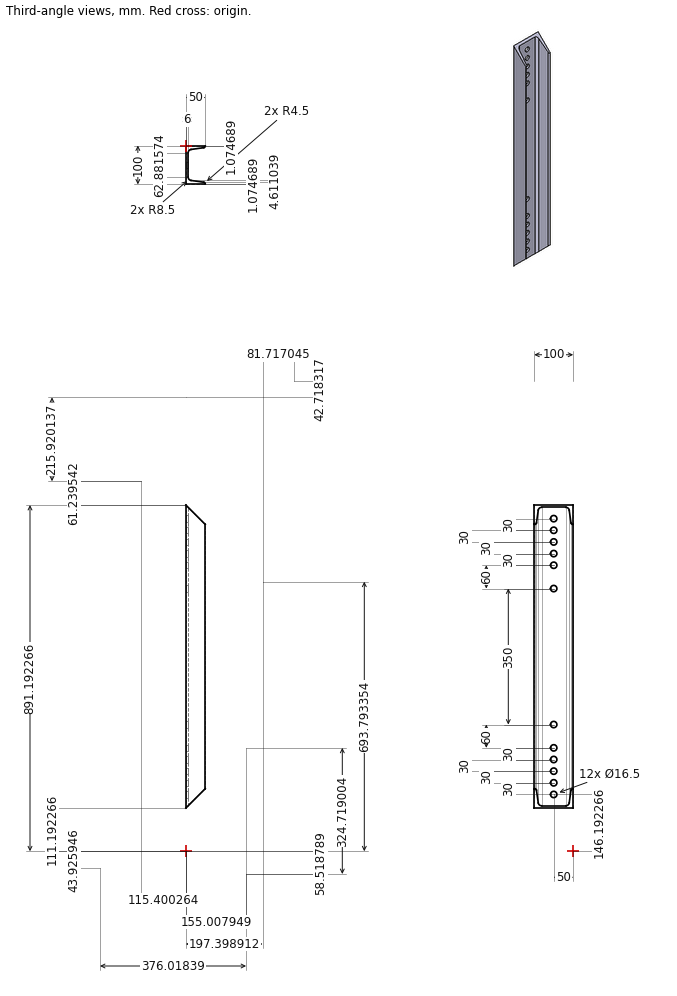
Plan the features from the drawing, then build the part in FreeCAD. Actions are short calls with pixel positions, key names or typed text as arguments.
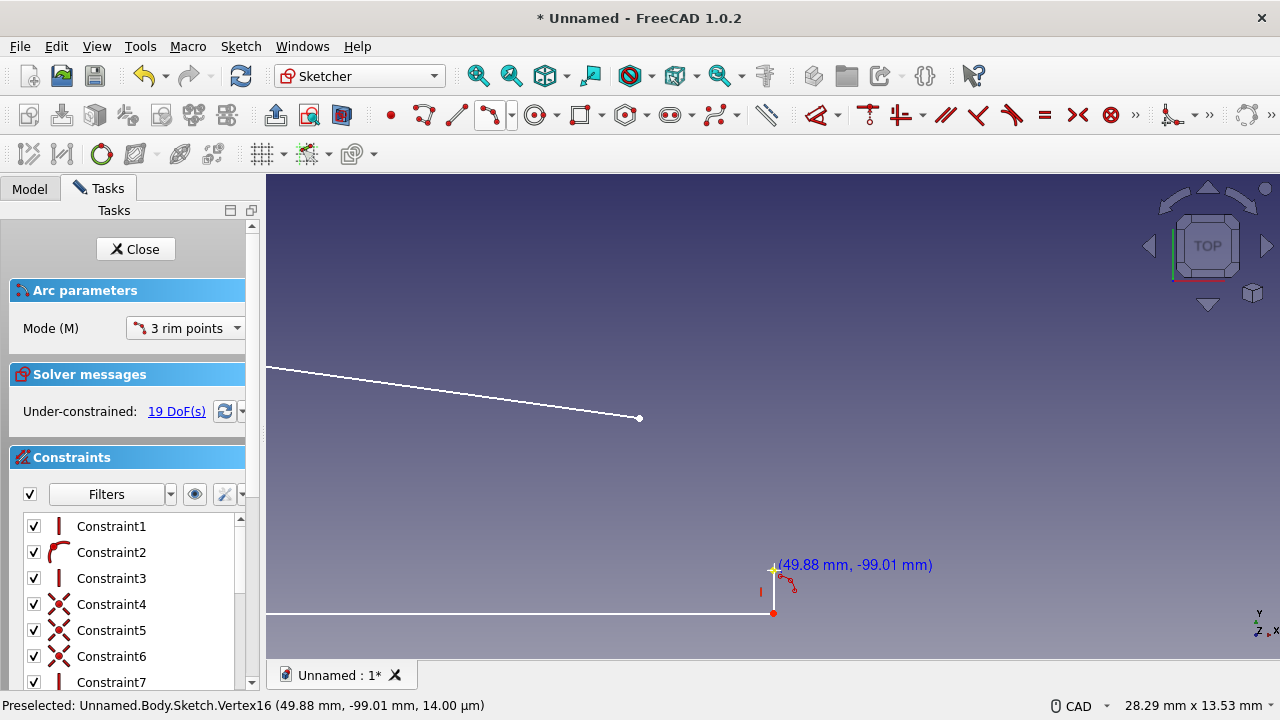
scroll(787, 576, down, 12)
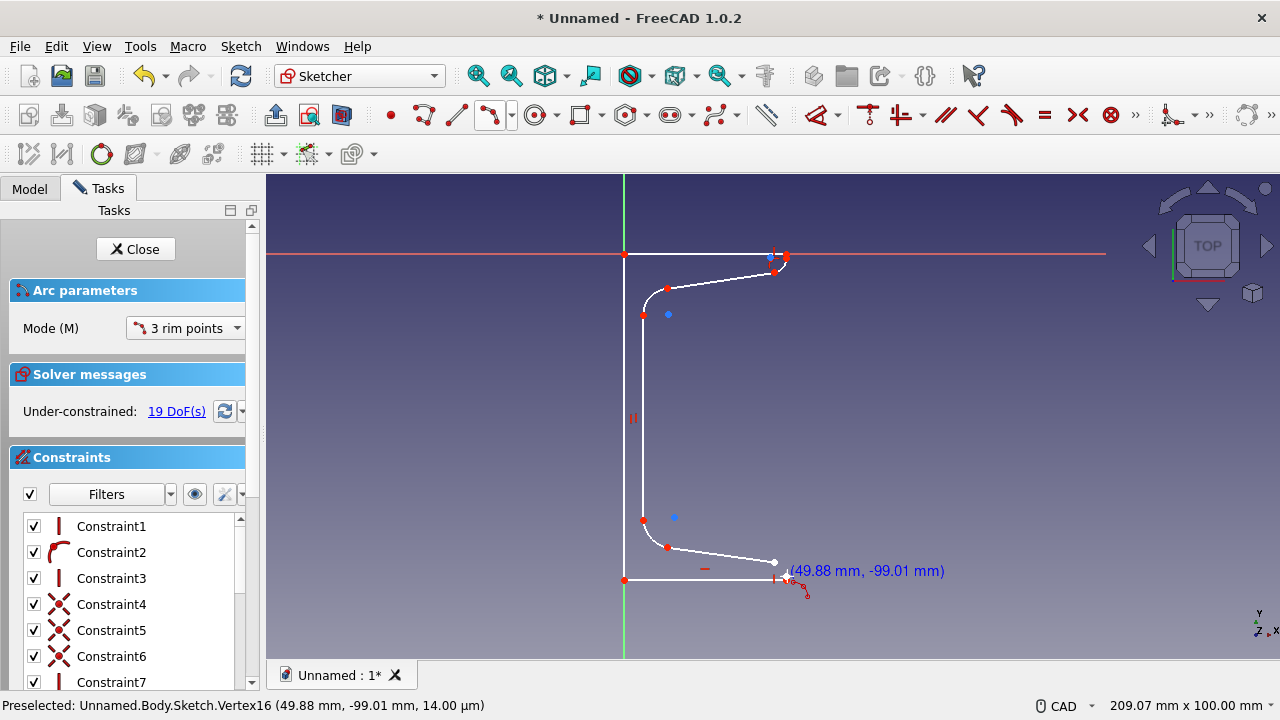
click(774, 562)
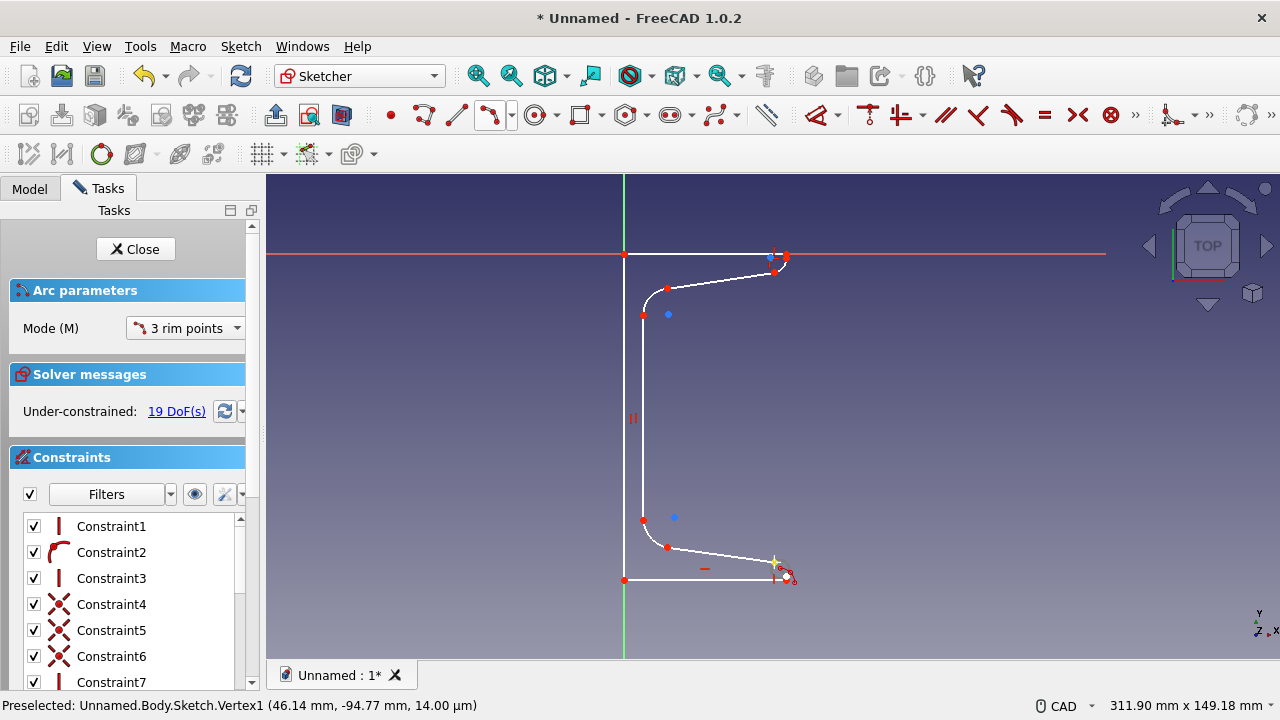
scroll(783, 566, up, 8)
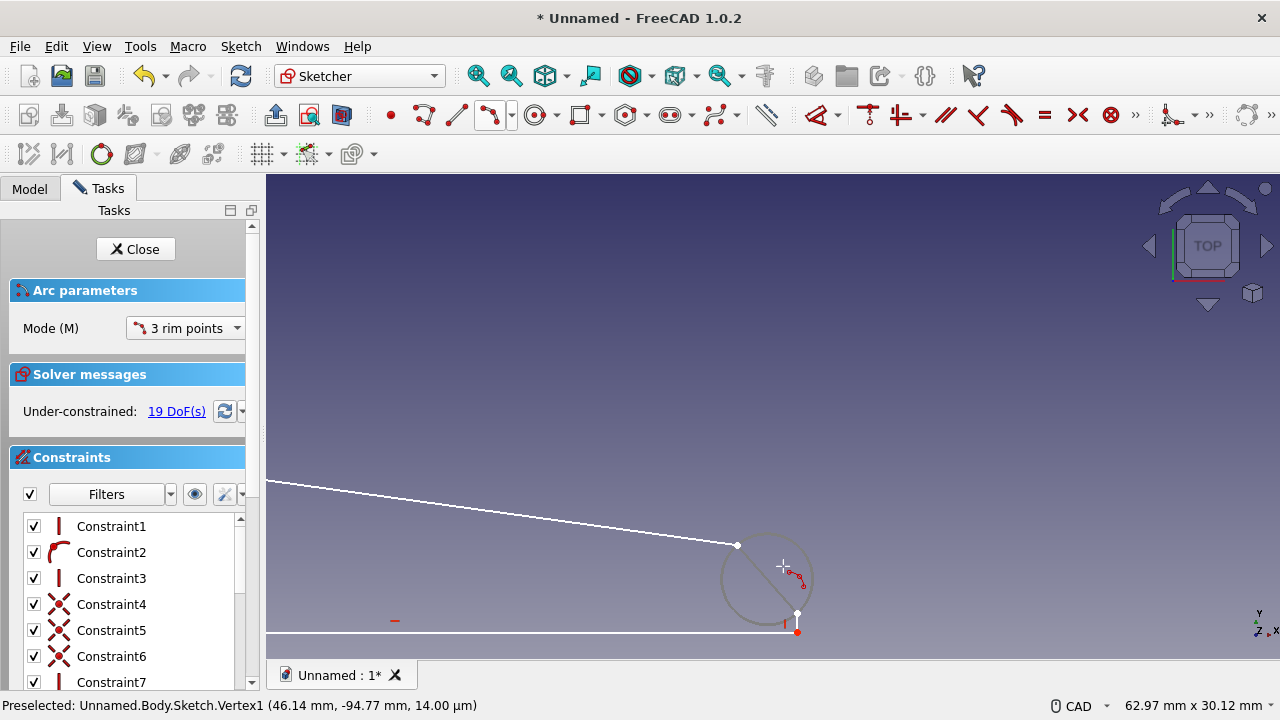
click(781, 565)
key(Escape)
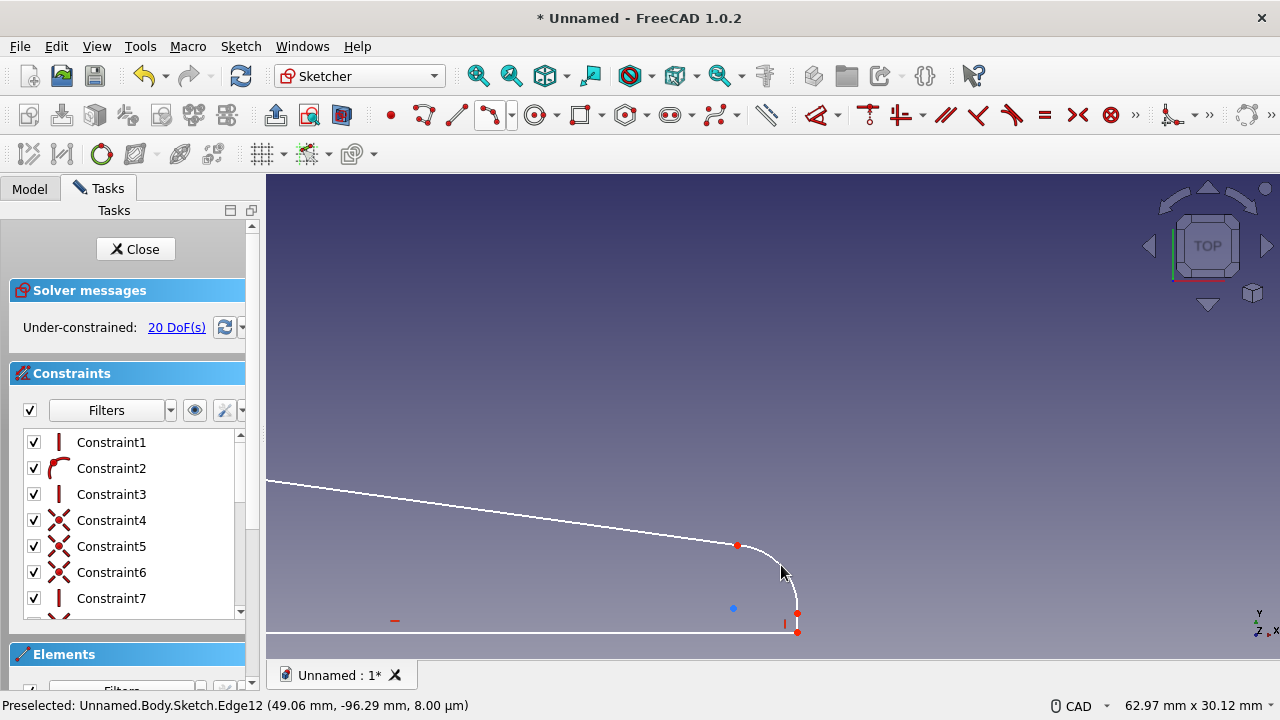
scroll(782, 566, down, 8)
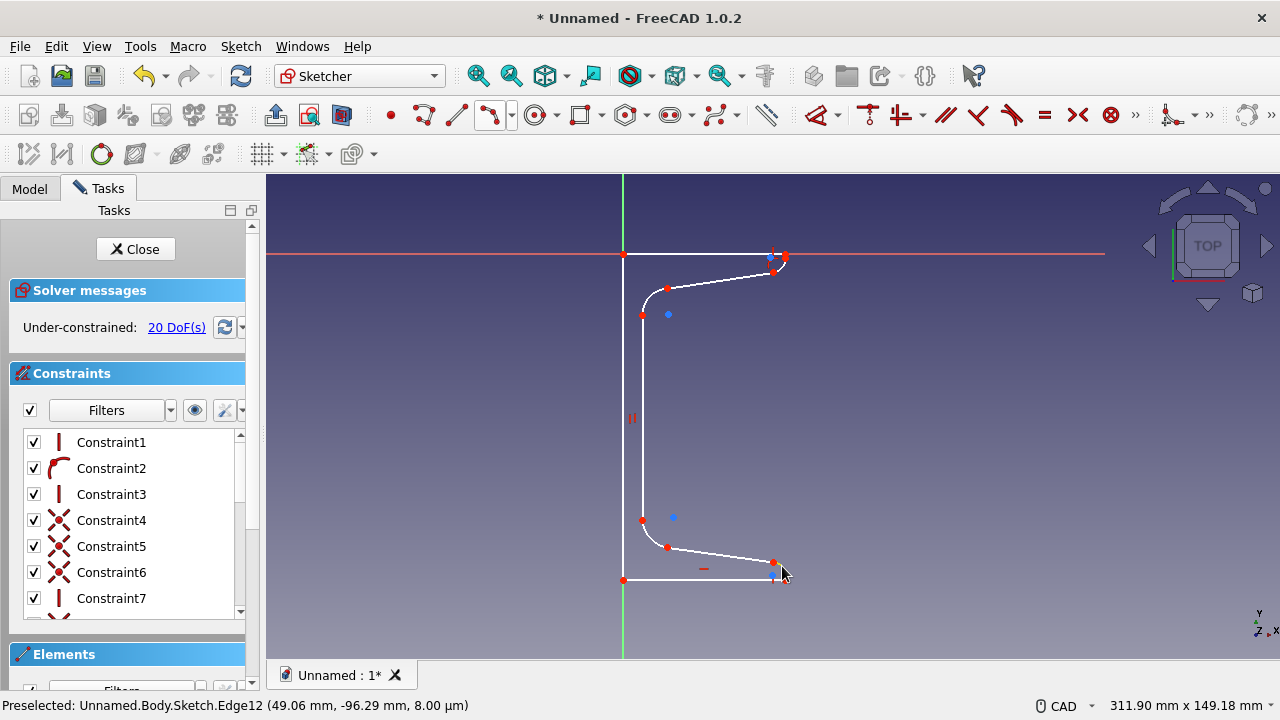
click(741, 558)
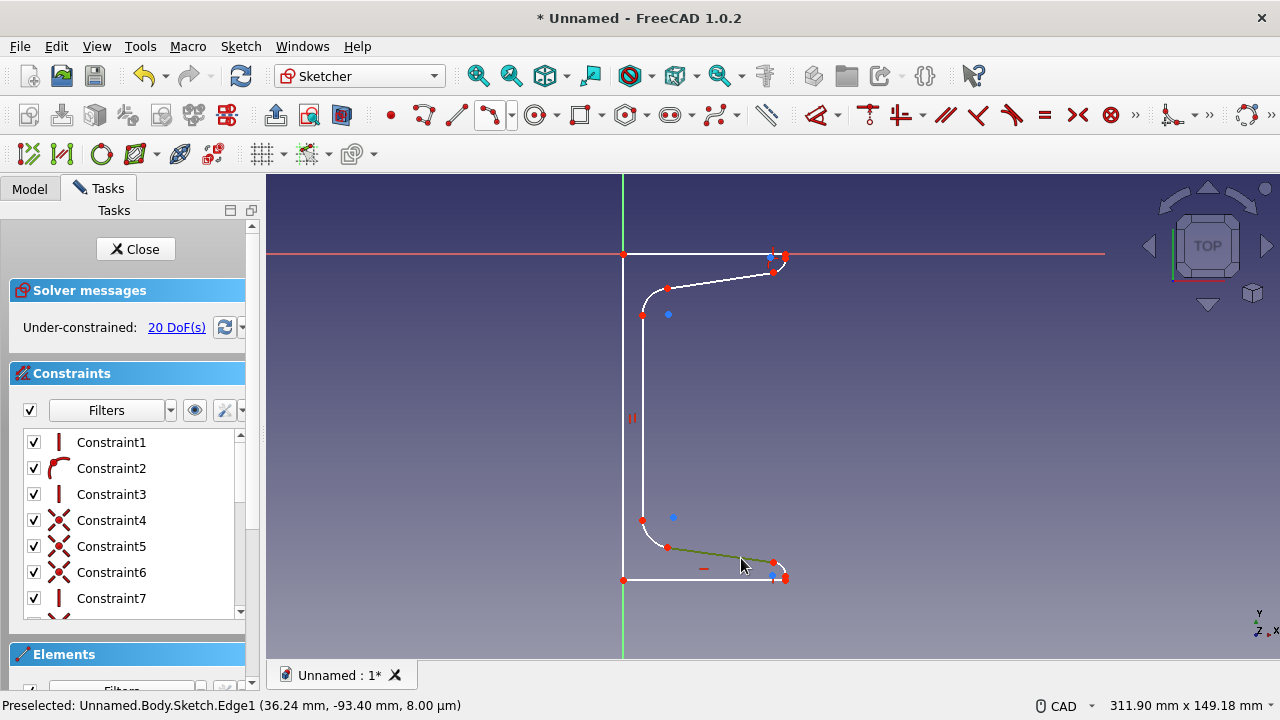
click(646, 532)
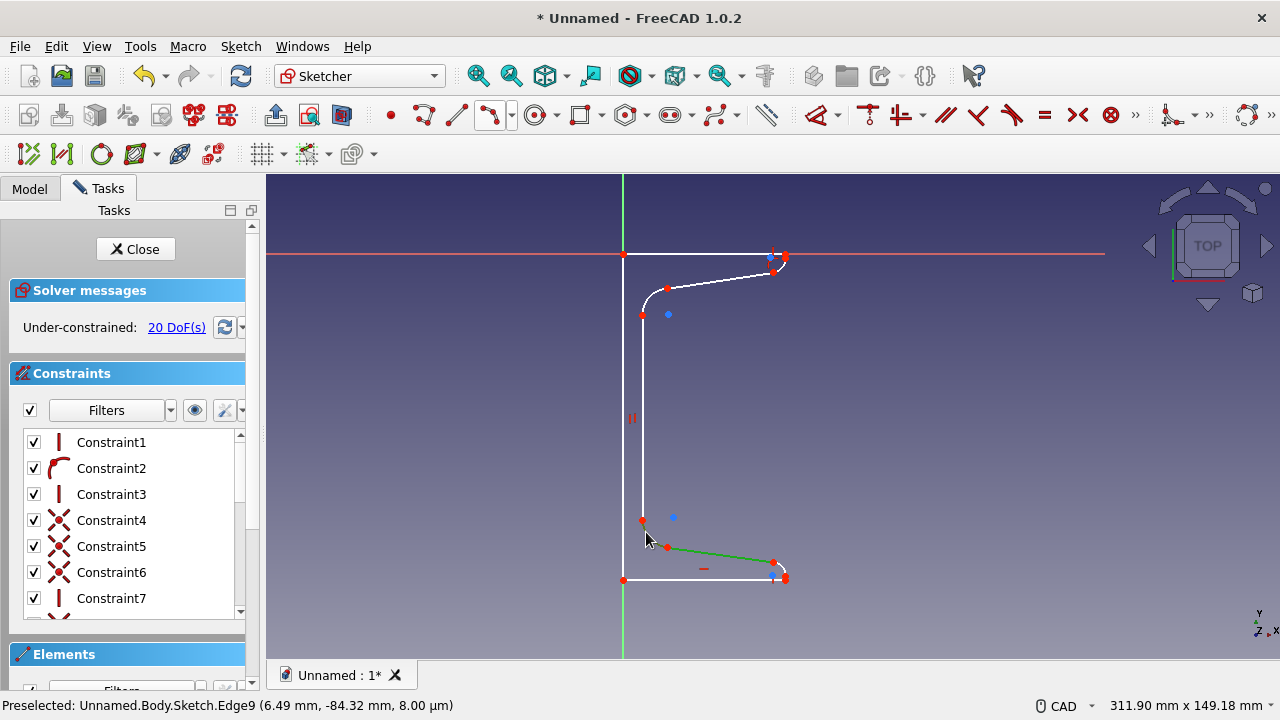
click(1012, 116)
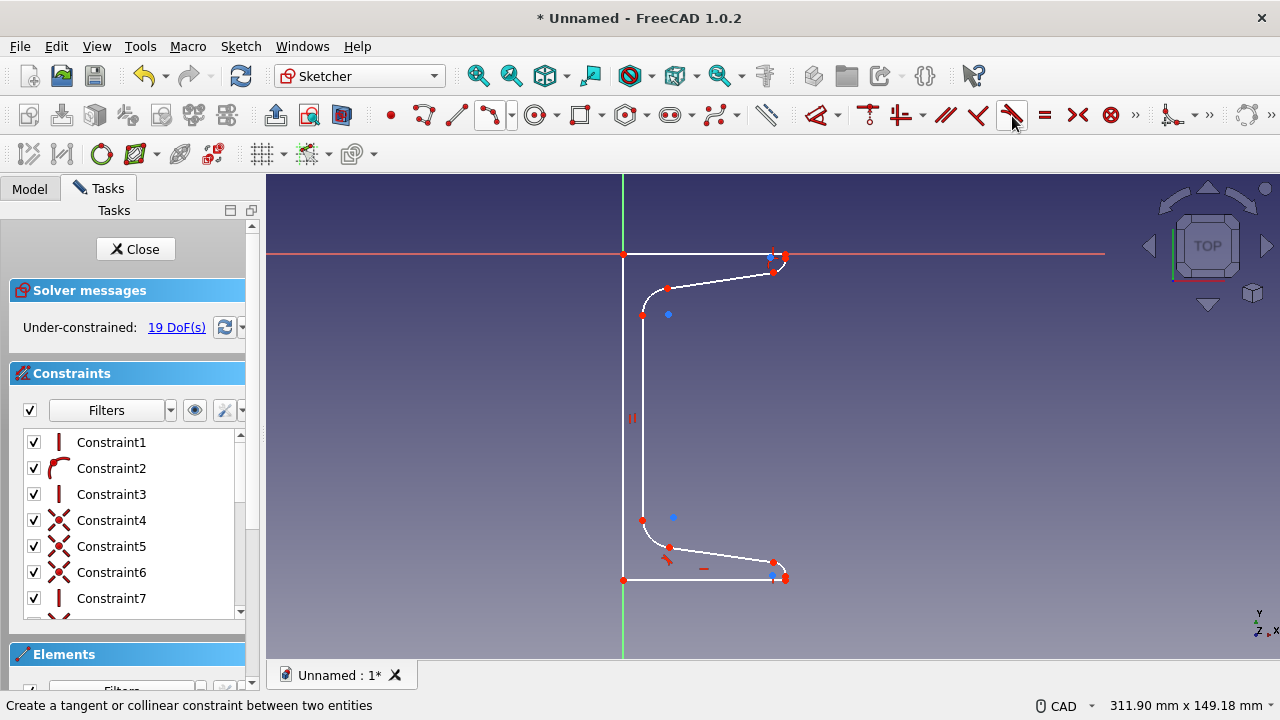
click(742, 558)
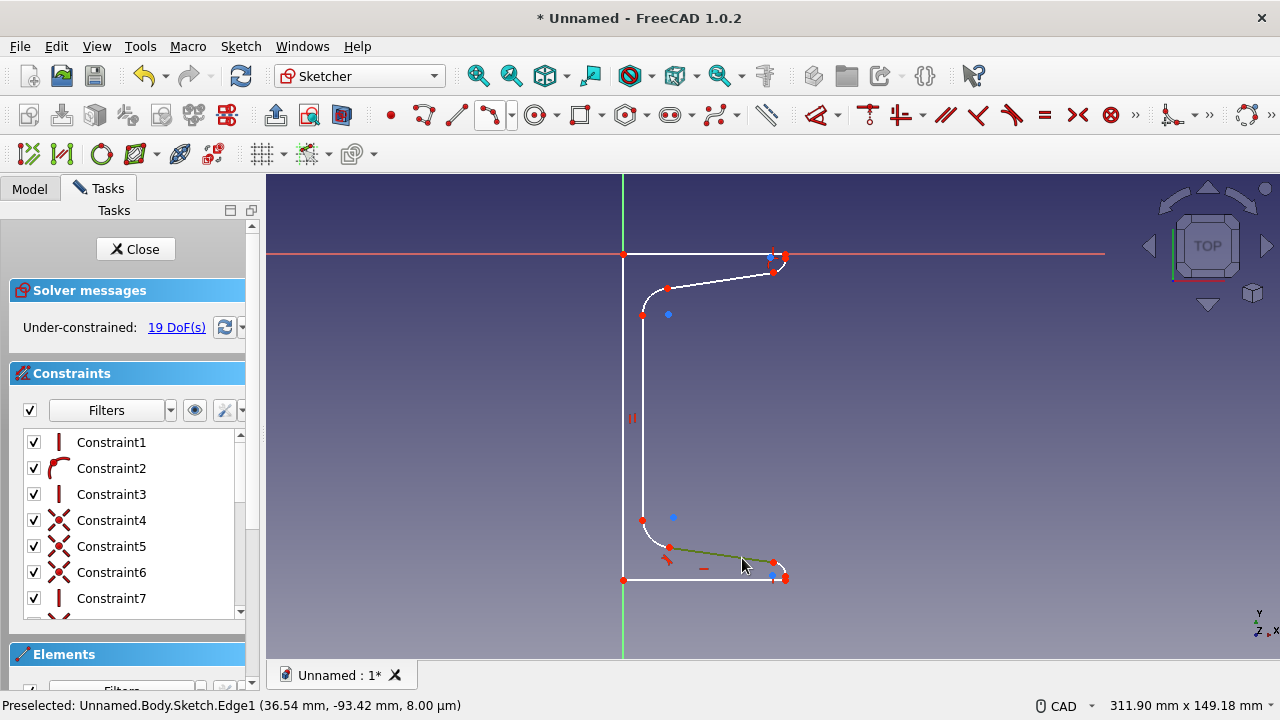
scroll(782, 567, up, 2)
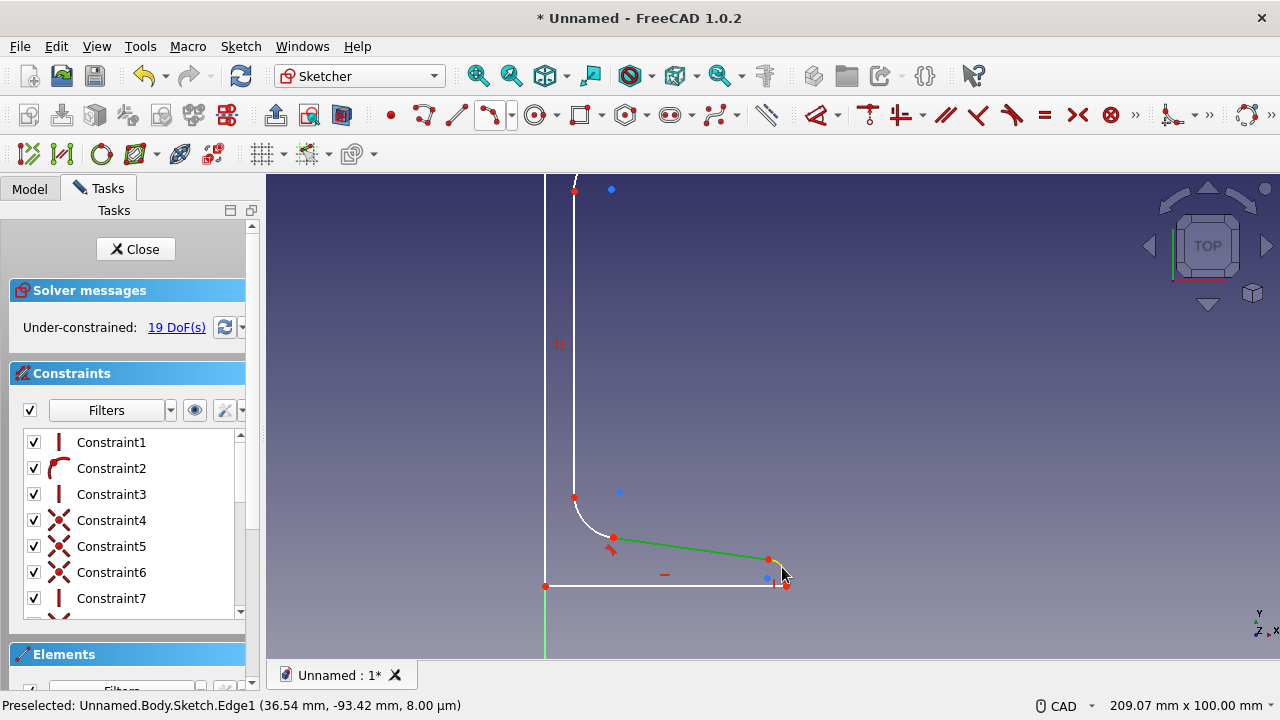
click(782, 566)